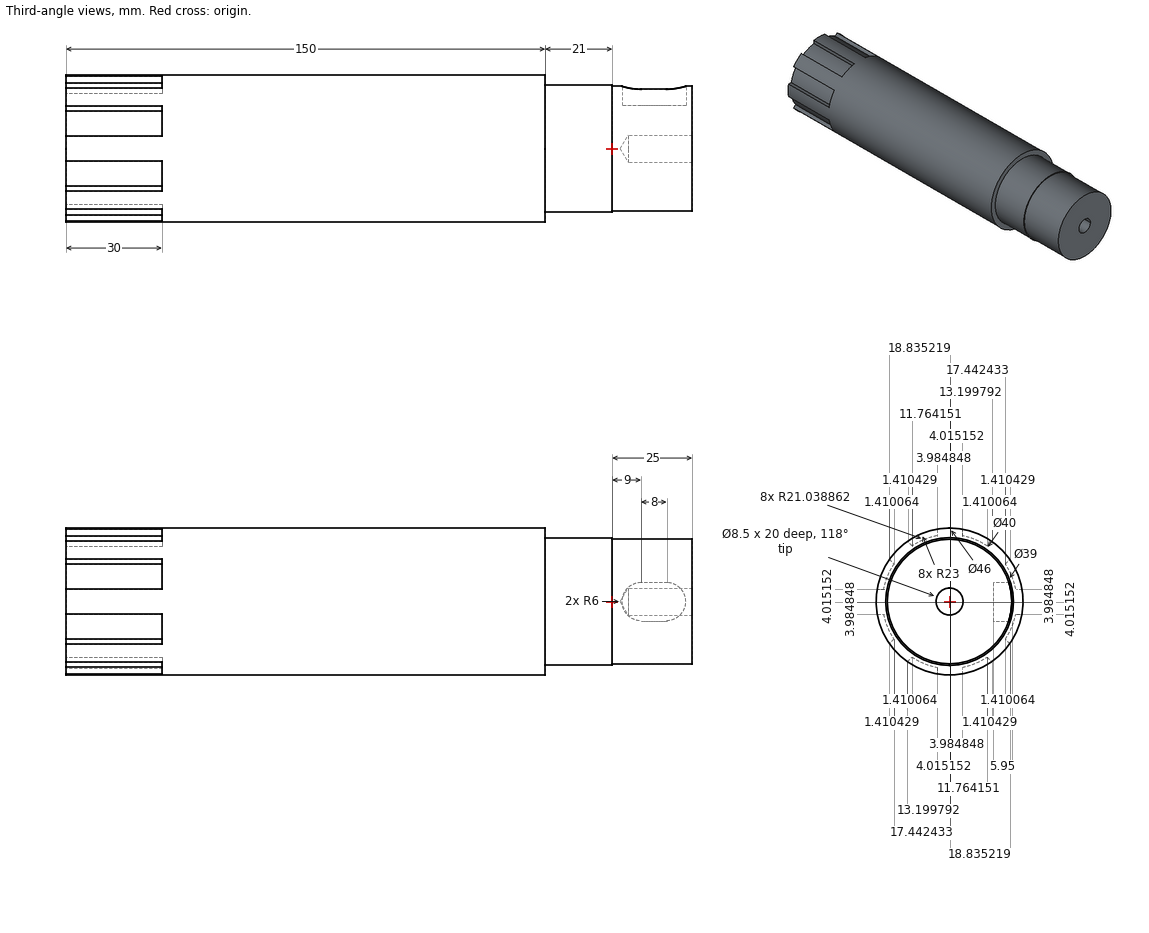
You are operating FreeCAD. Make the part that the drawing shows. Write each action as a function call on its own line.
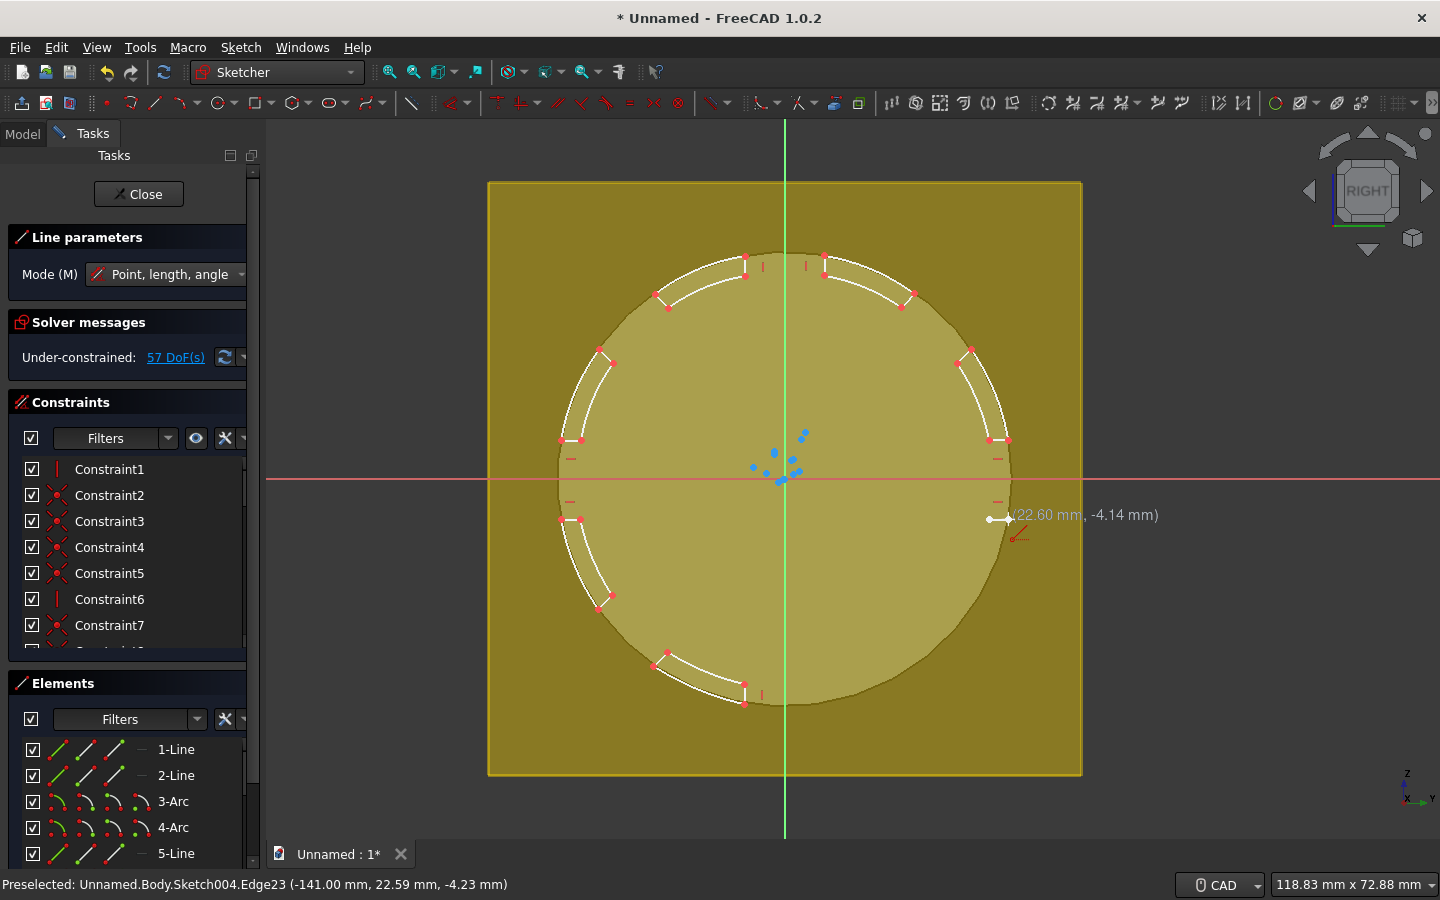
click(971, 610)
click(957, 596)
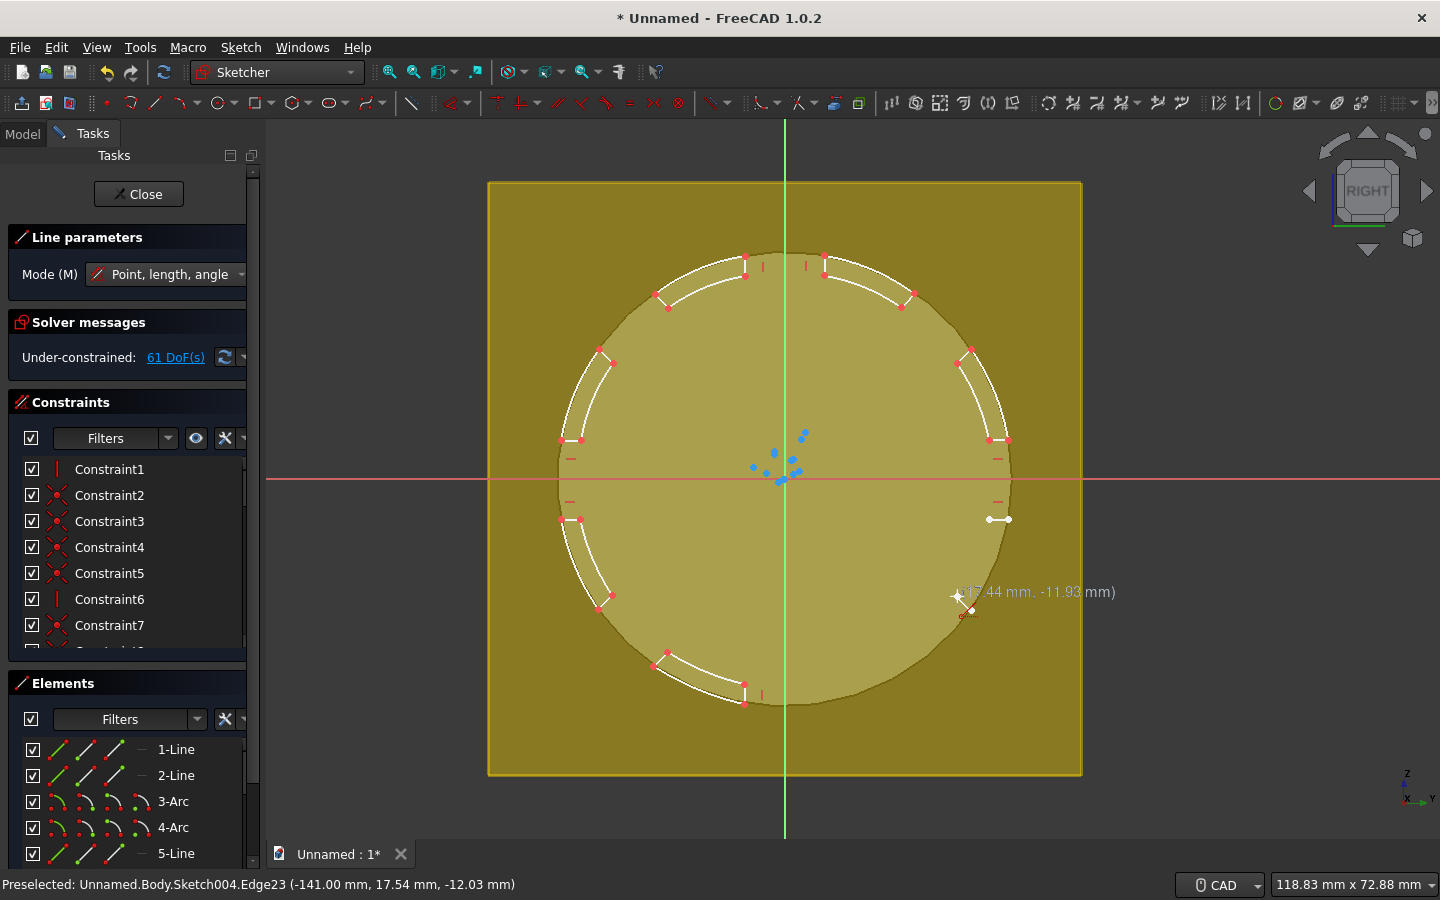
click(180, 104)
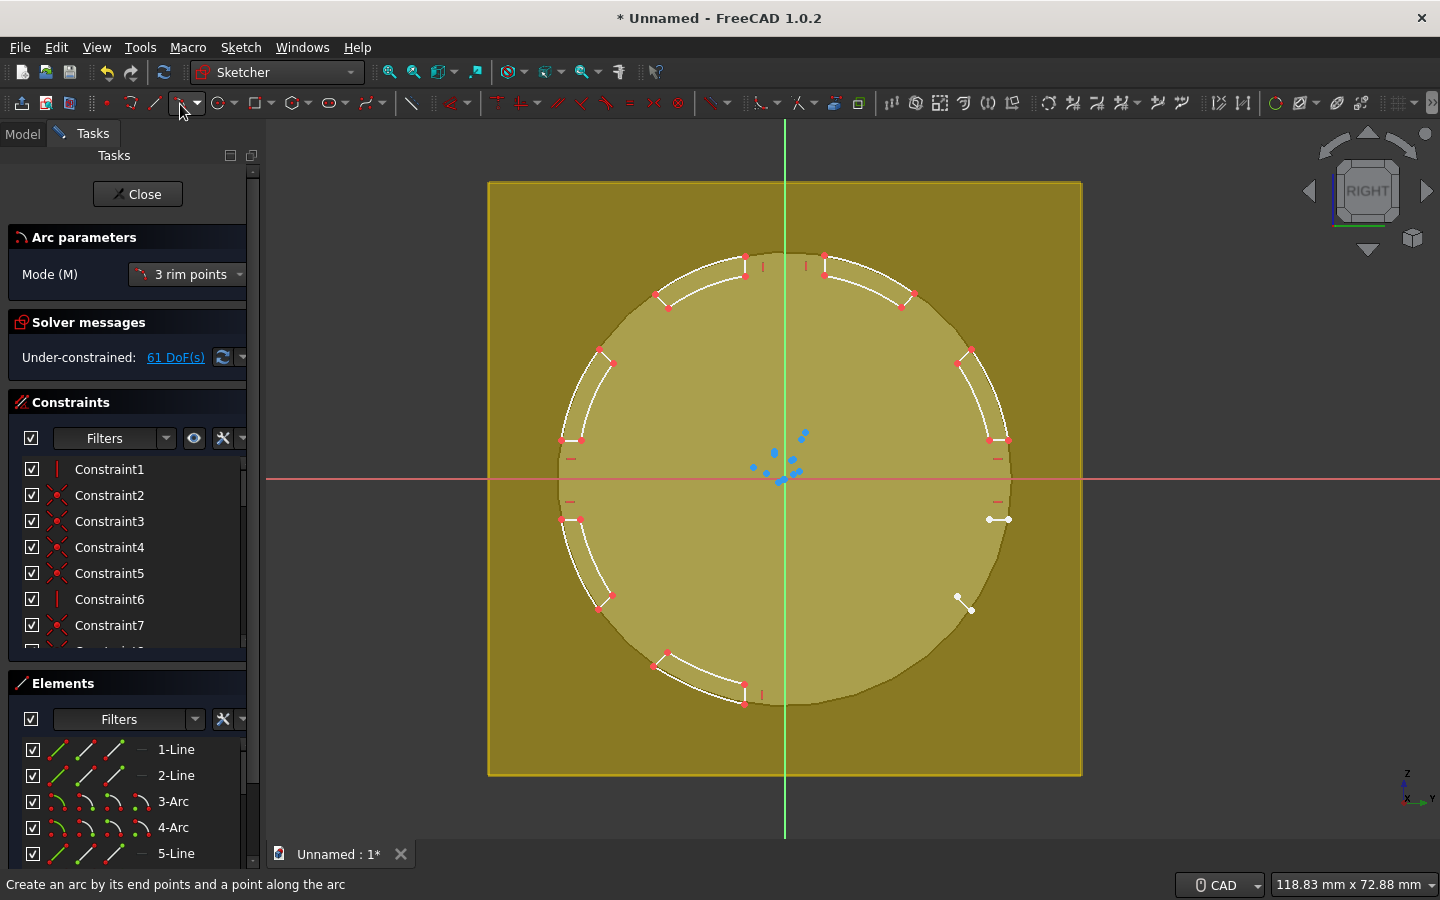
scroll(1008, 519, up, 3)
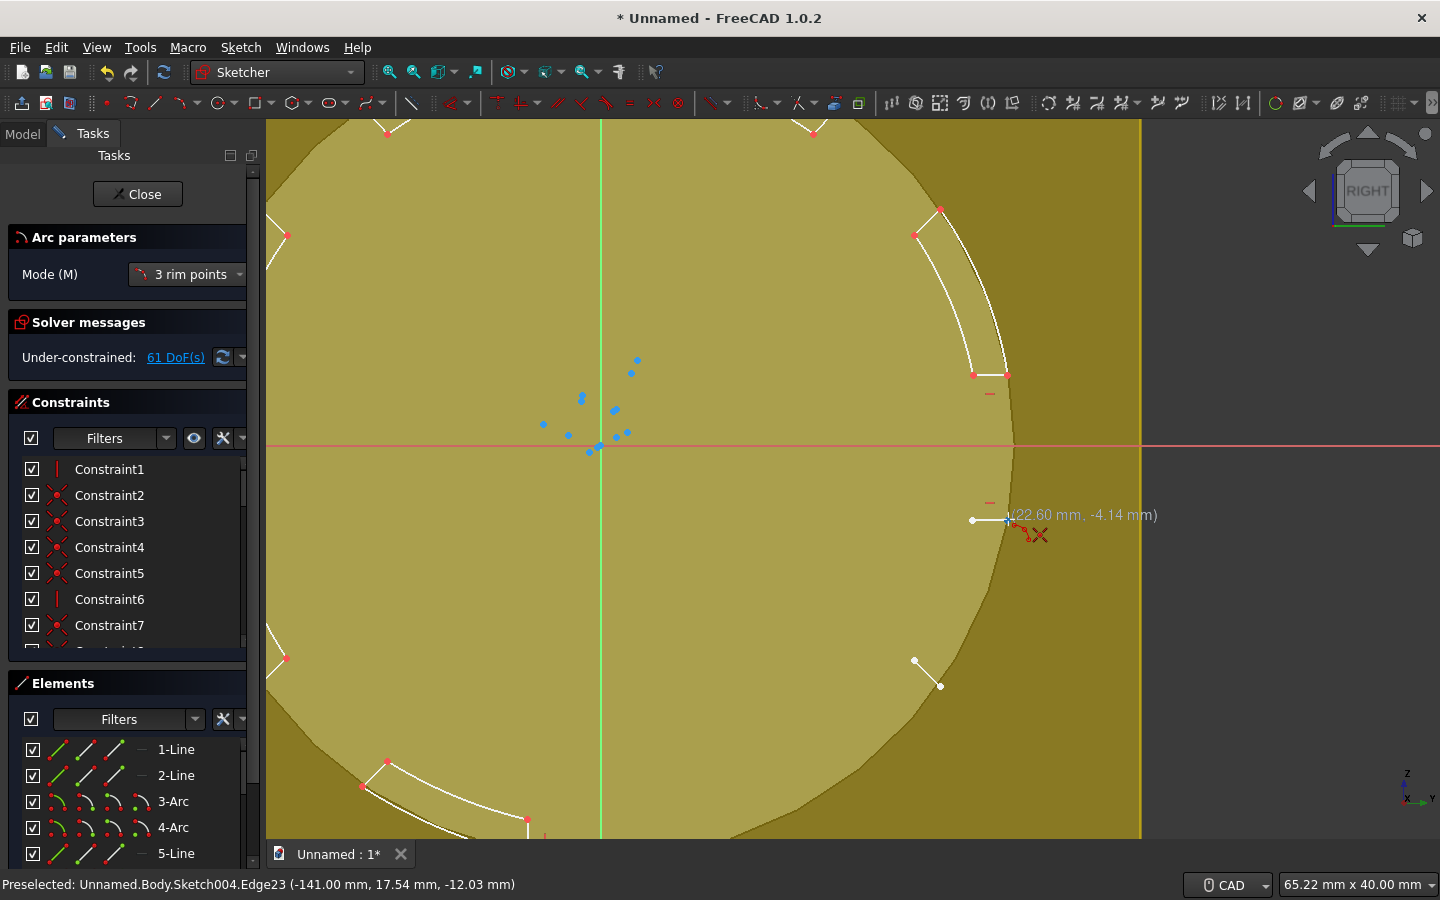
click(1007, 520)
click(940, 686)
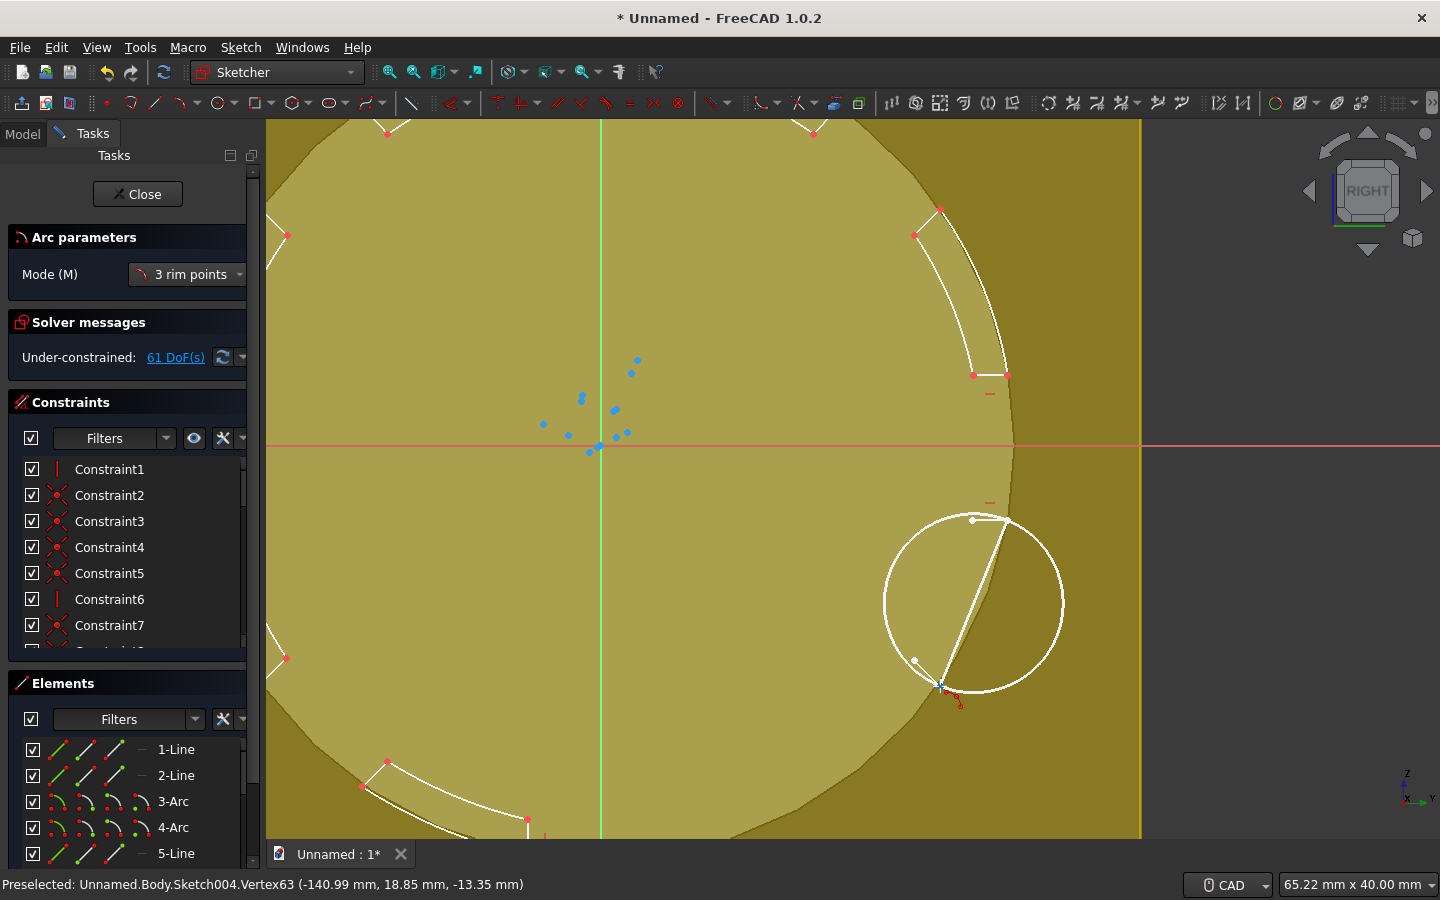
scroll(983, 605, up, 3)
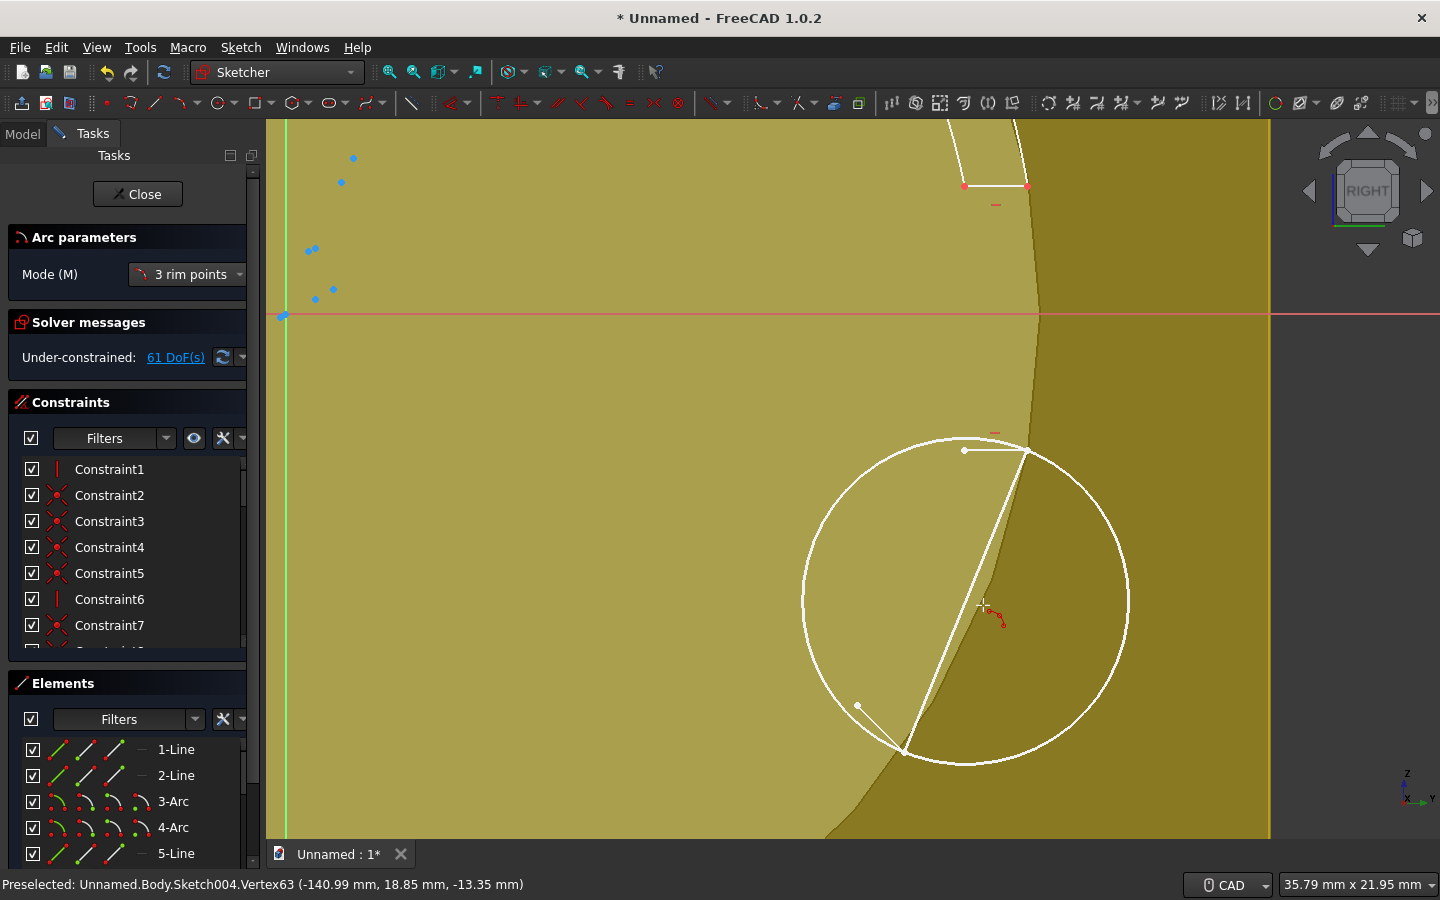
click(983, 604)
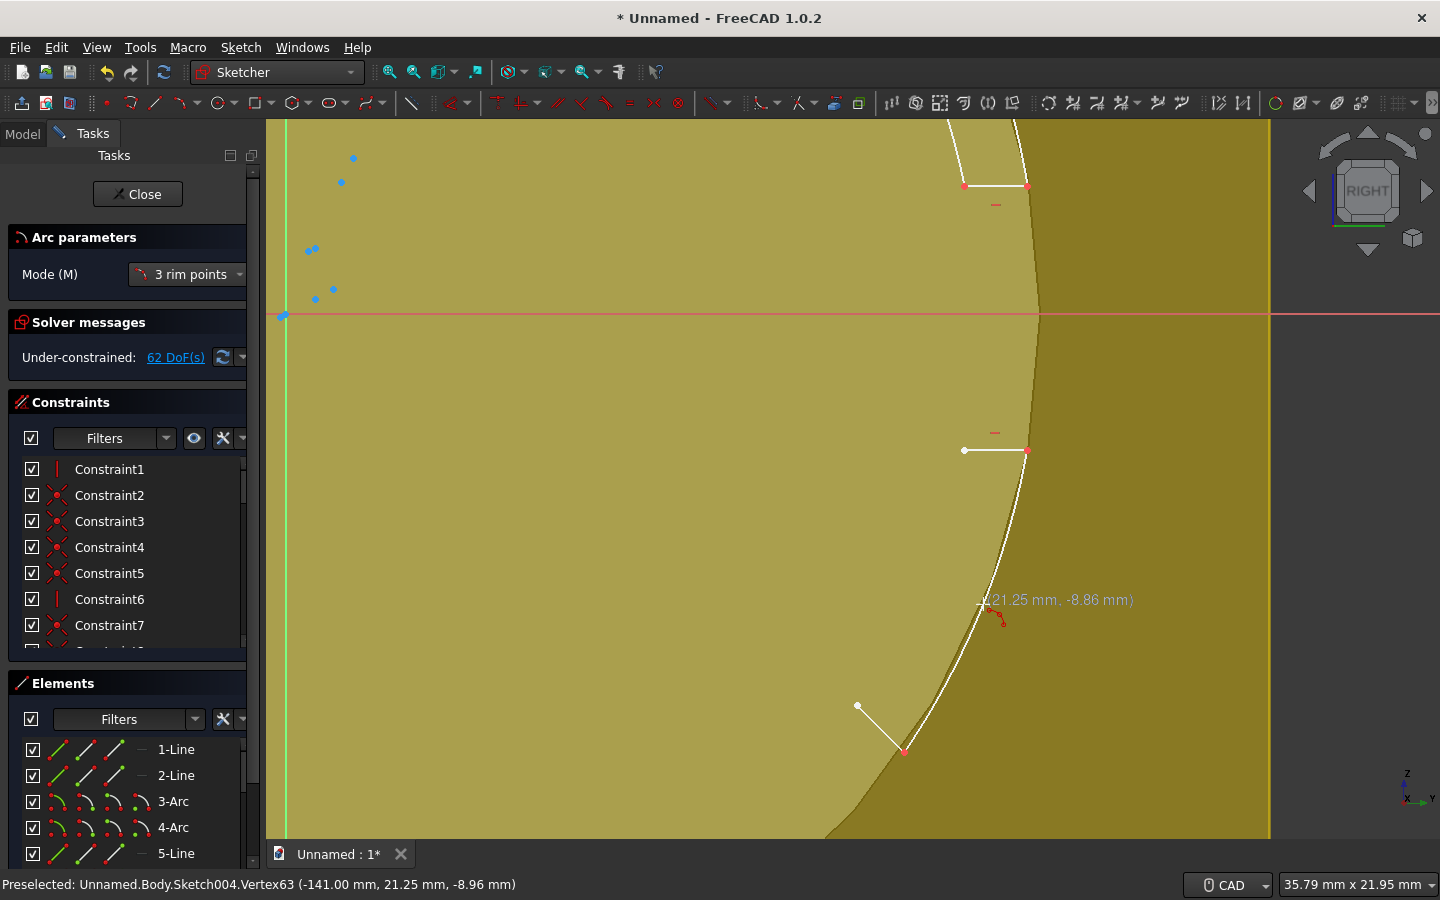
click(858, 706)
click(964, 450)
click(923, 579)